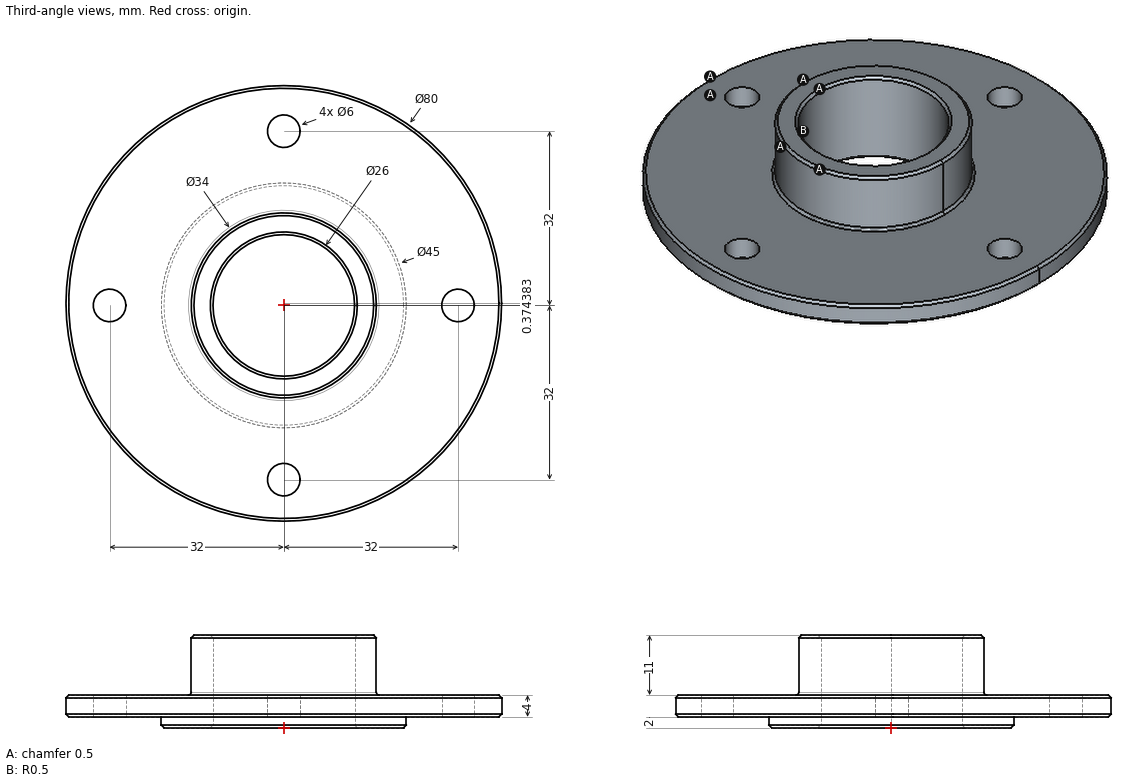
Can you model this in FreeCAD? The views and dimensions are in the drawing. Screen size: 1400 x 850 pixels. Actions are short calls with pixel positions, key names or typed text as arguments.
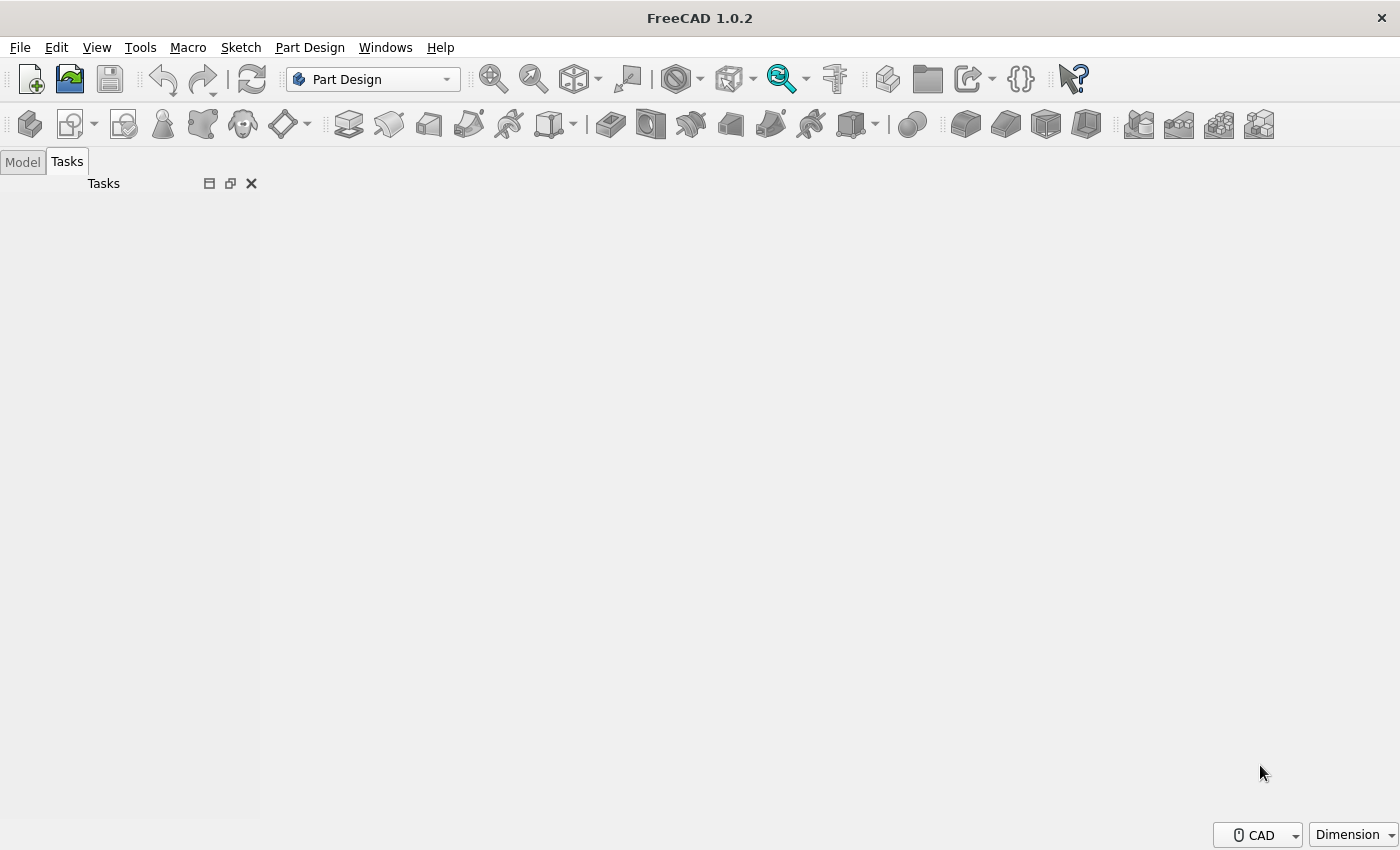
click(30, 80)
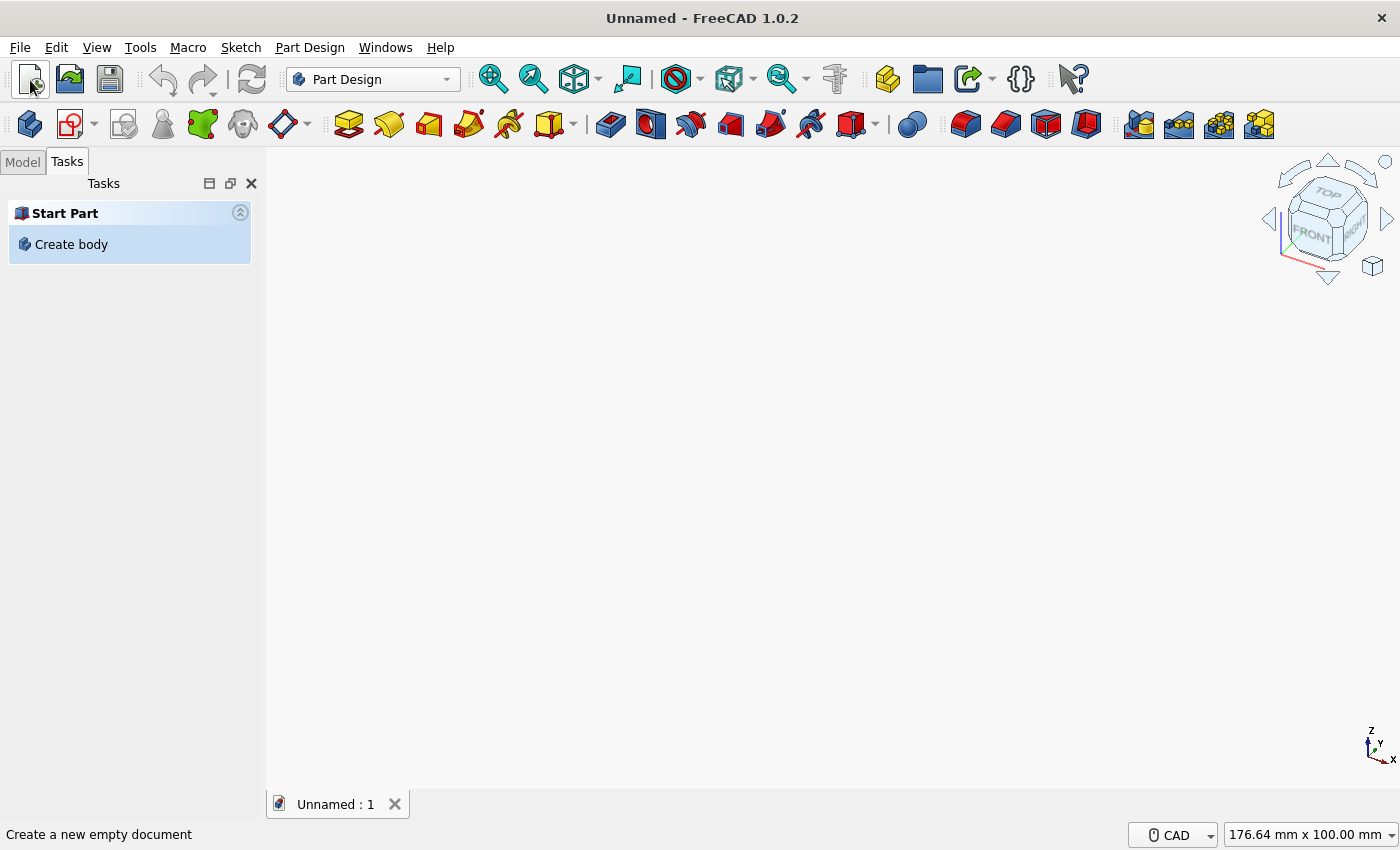
click(70, 124)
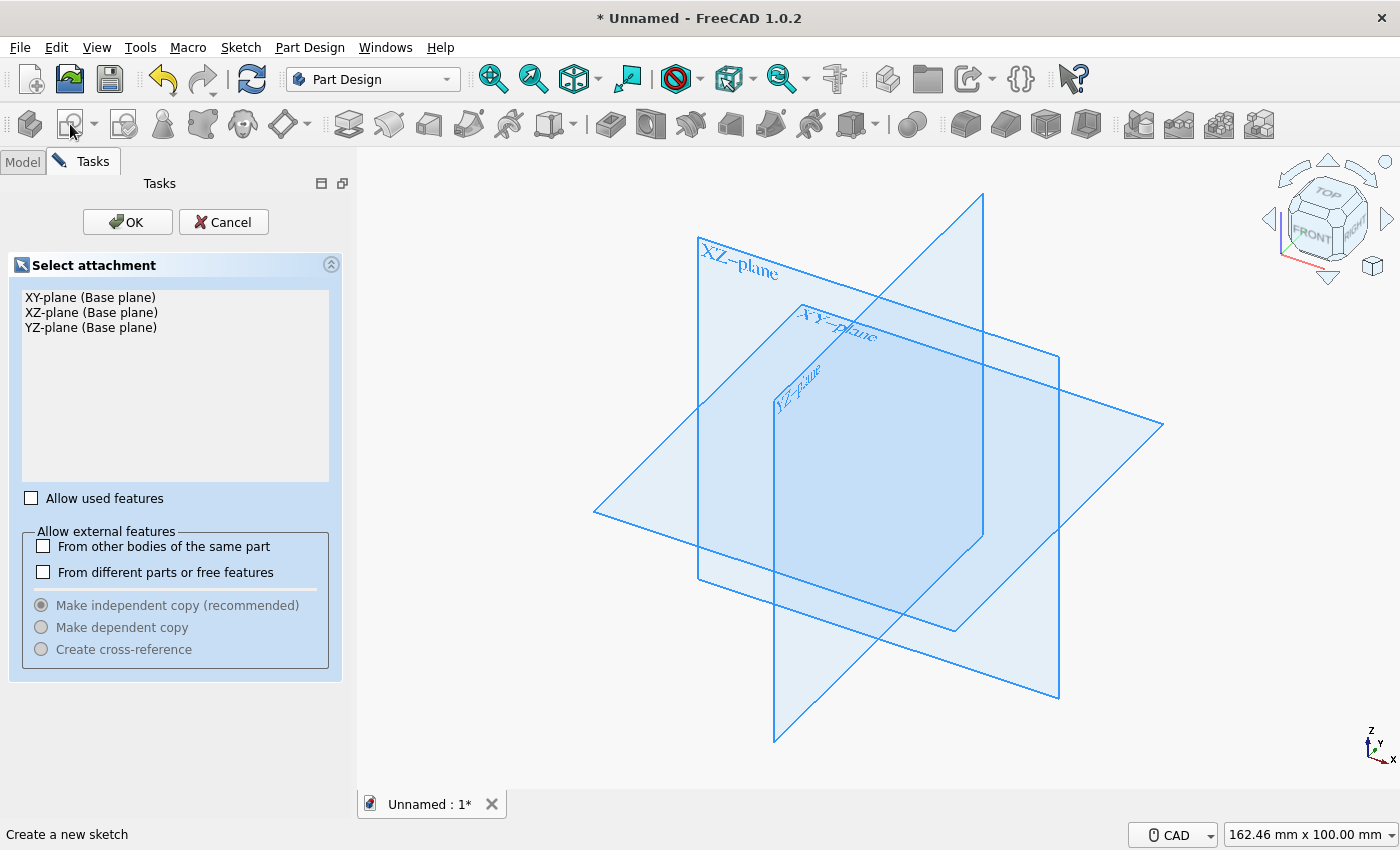
click(82, 298)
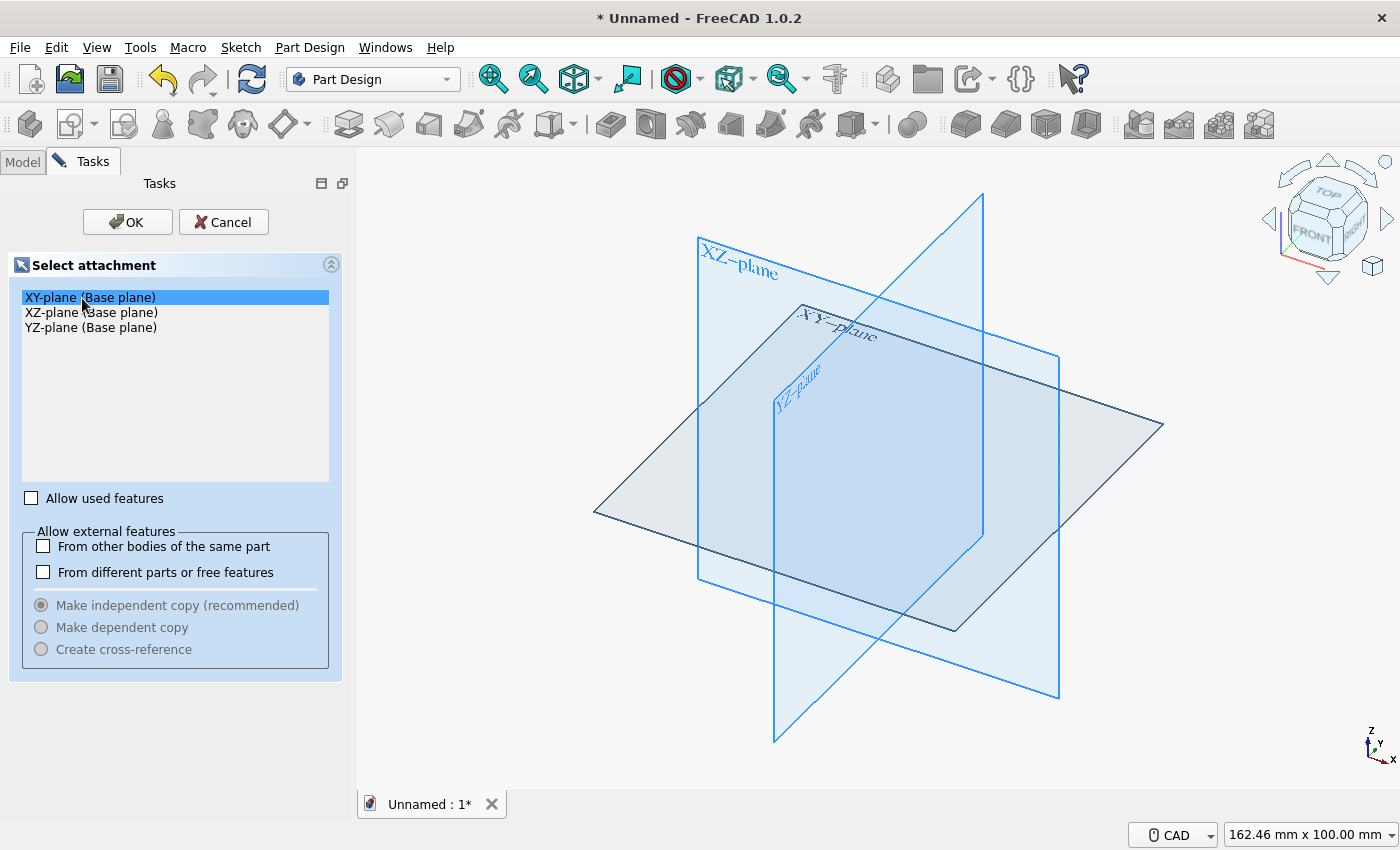
click(128, 222)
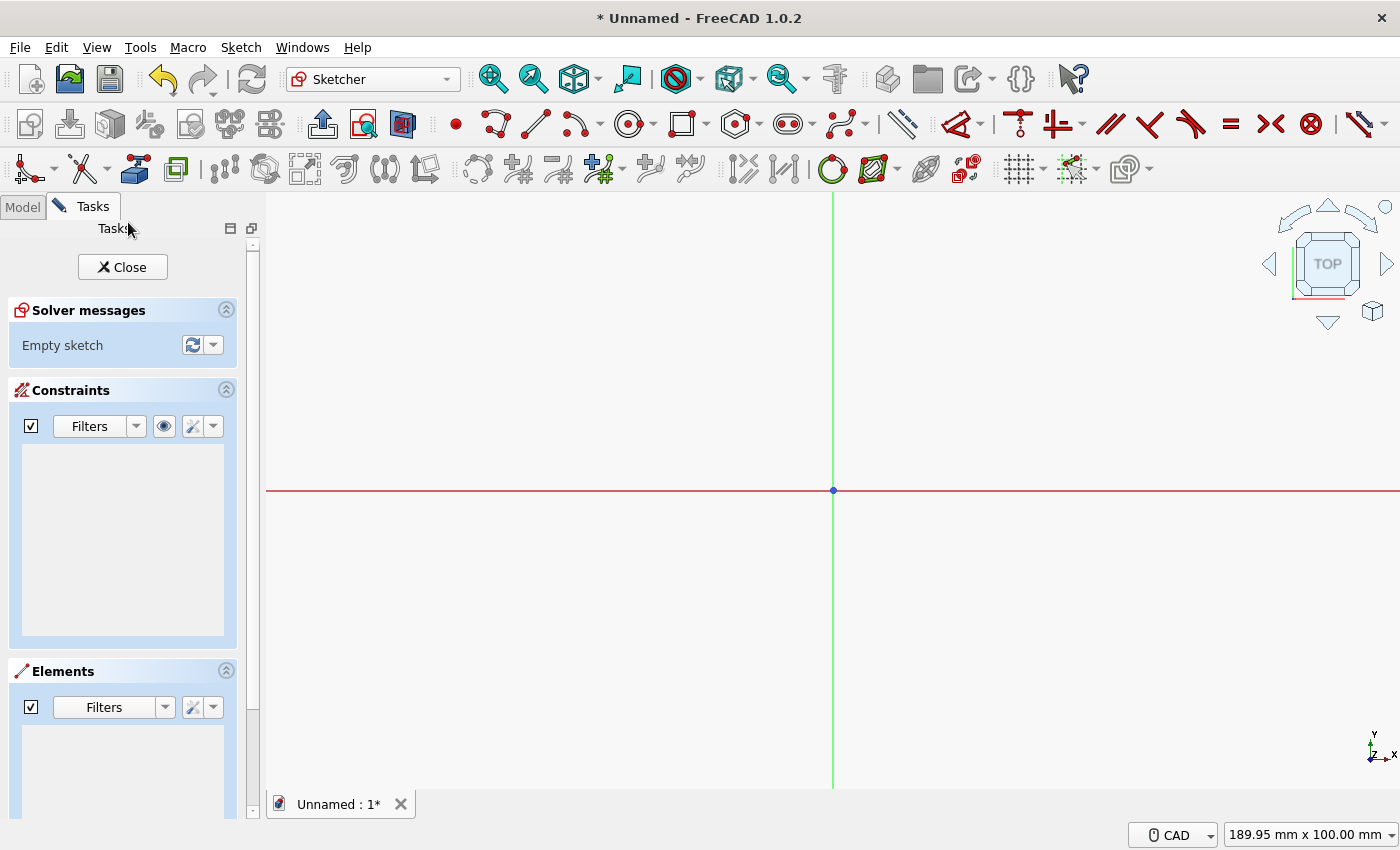
scroll(972, 490, up, 2)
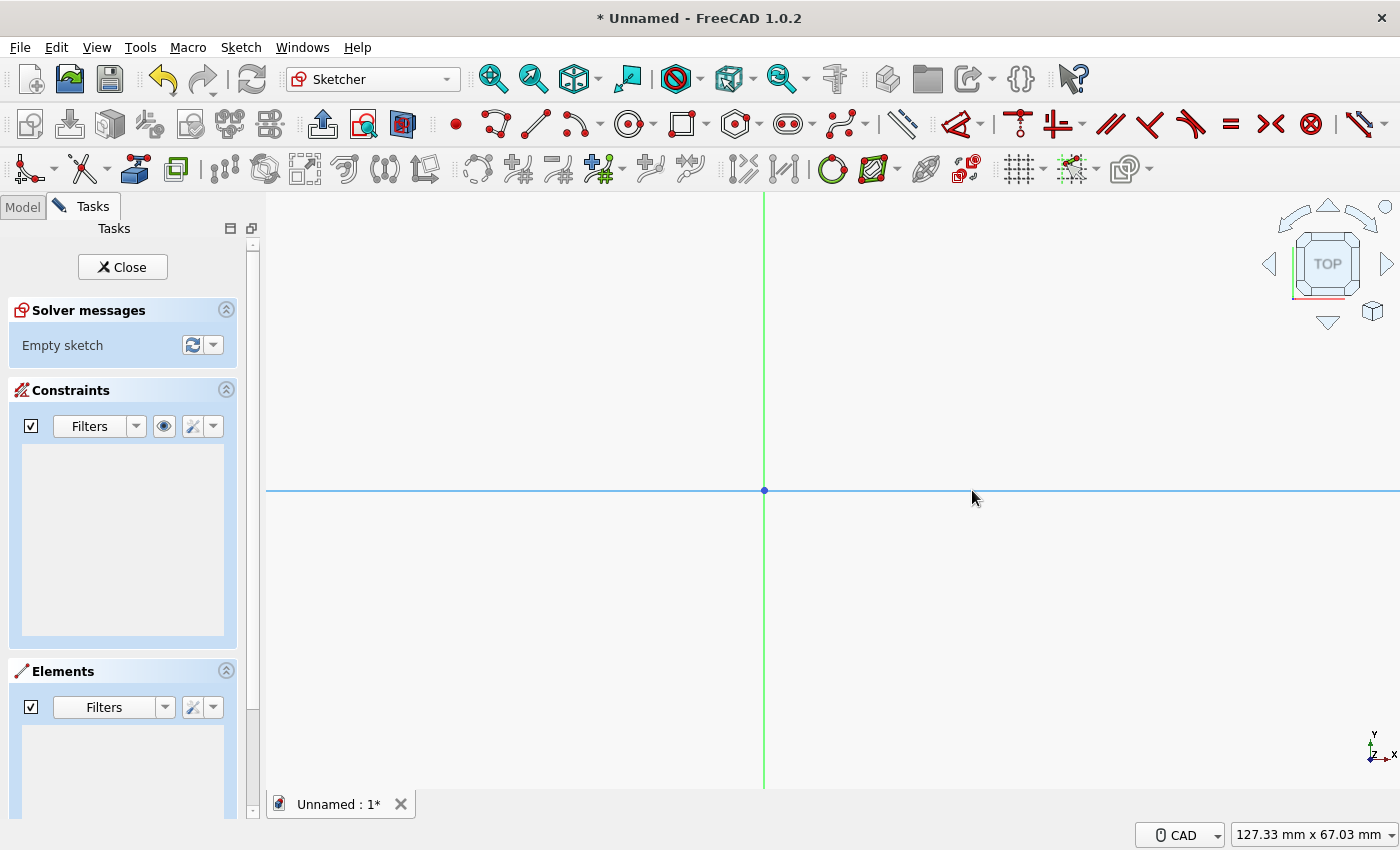
click(630, 124)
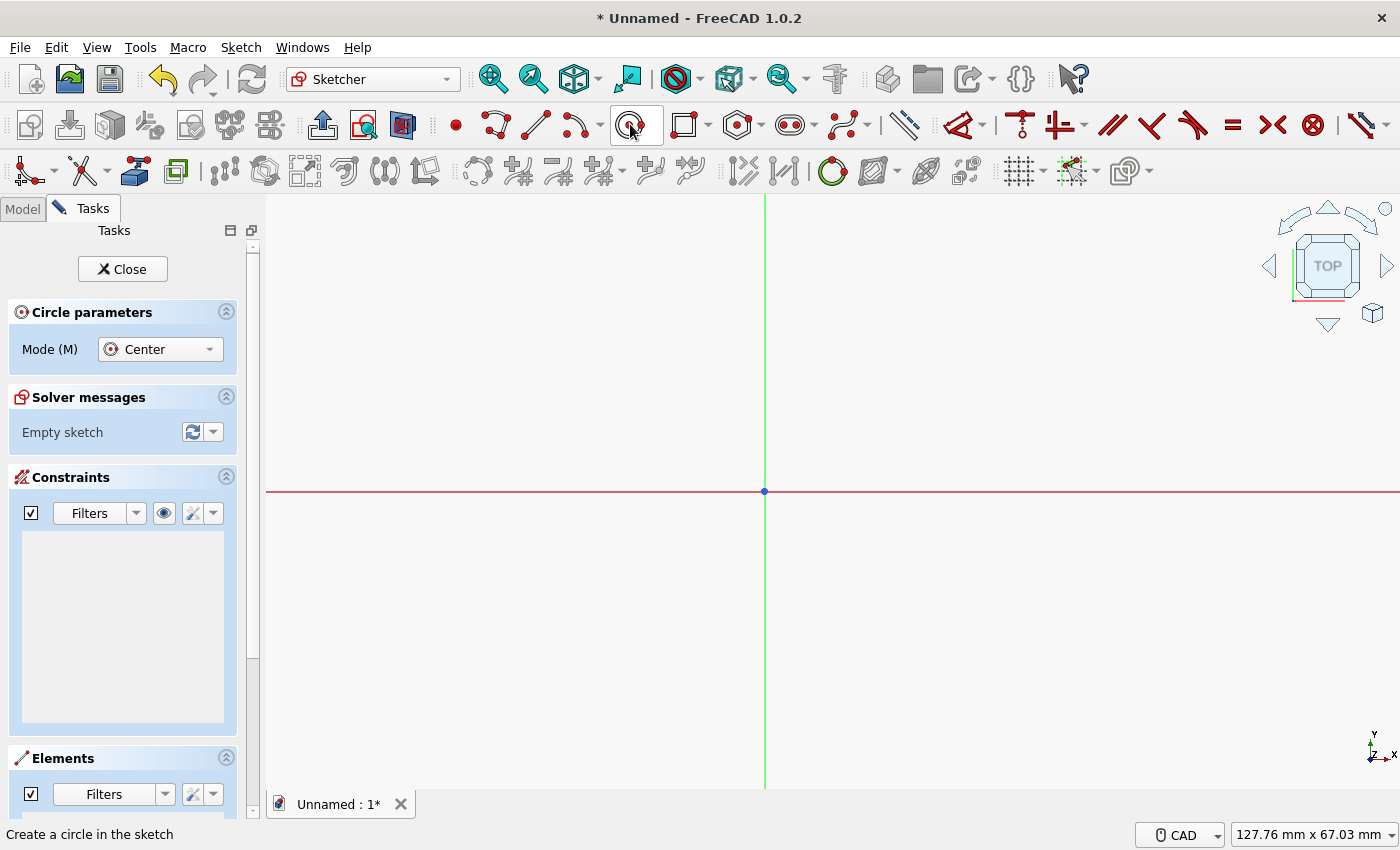
click(765, 492)
move(906, 350)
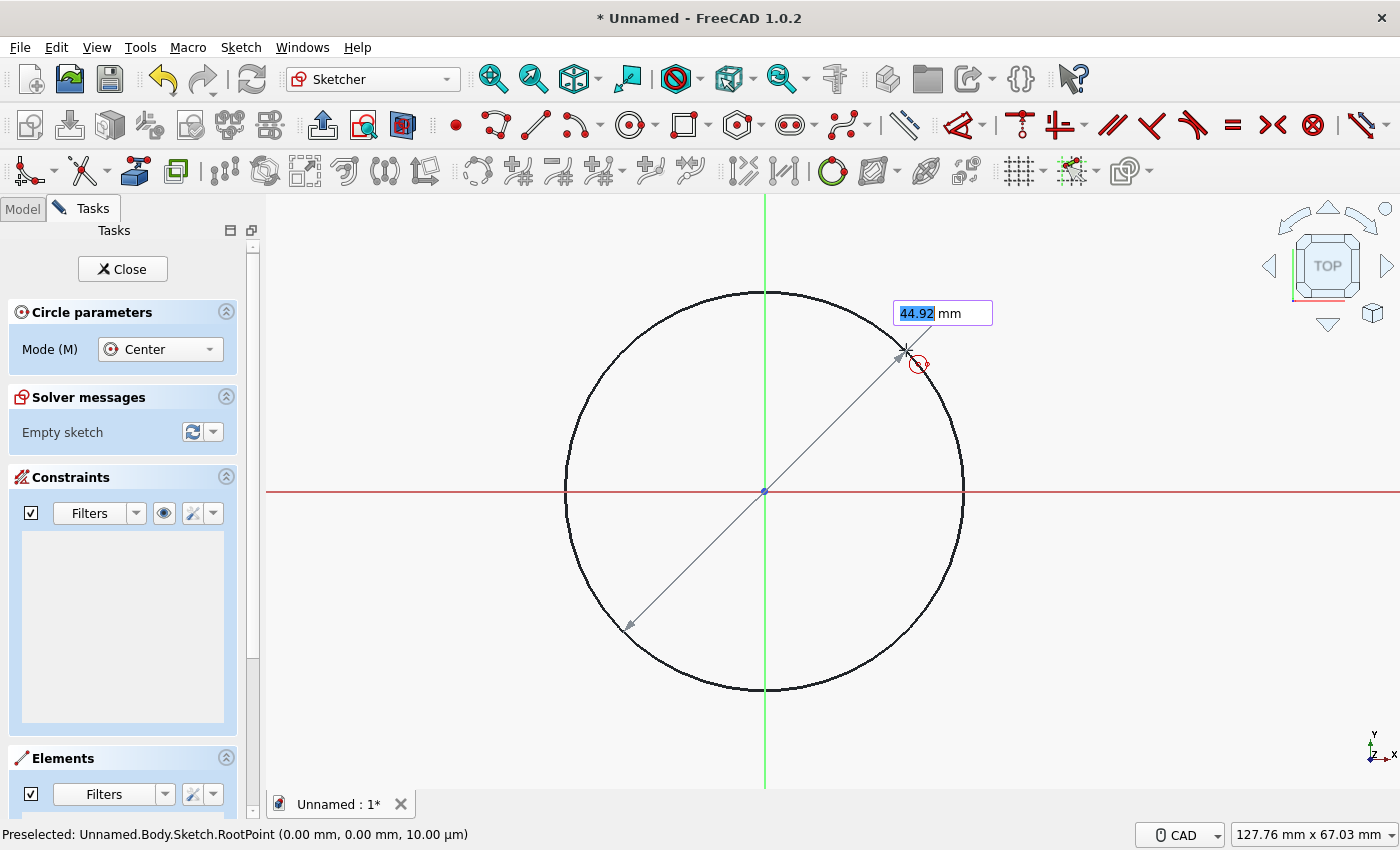
text(45)
key(Return)